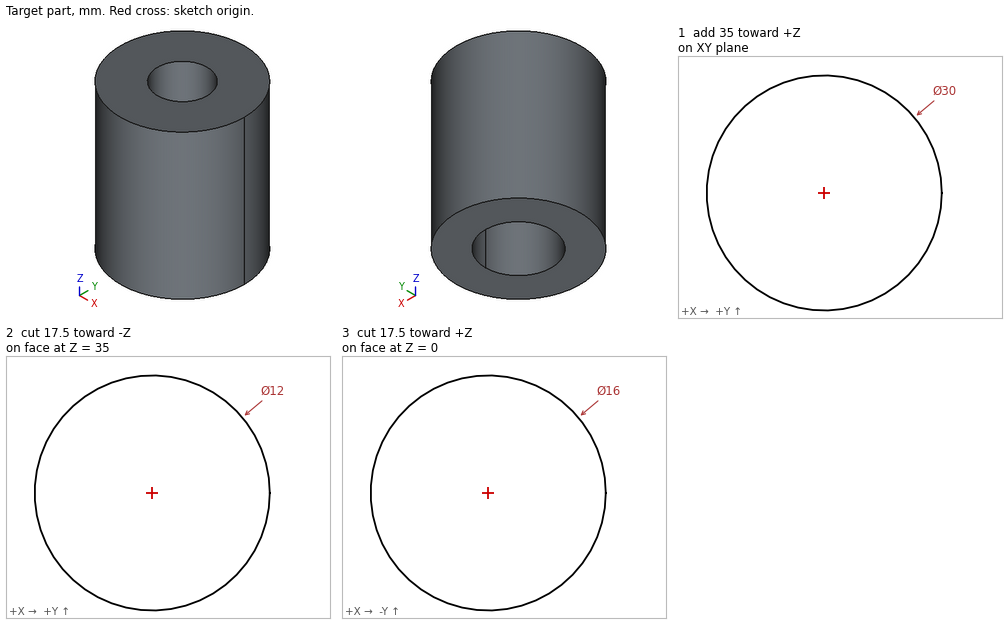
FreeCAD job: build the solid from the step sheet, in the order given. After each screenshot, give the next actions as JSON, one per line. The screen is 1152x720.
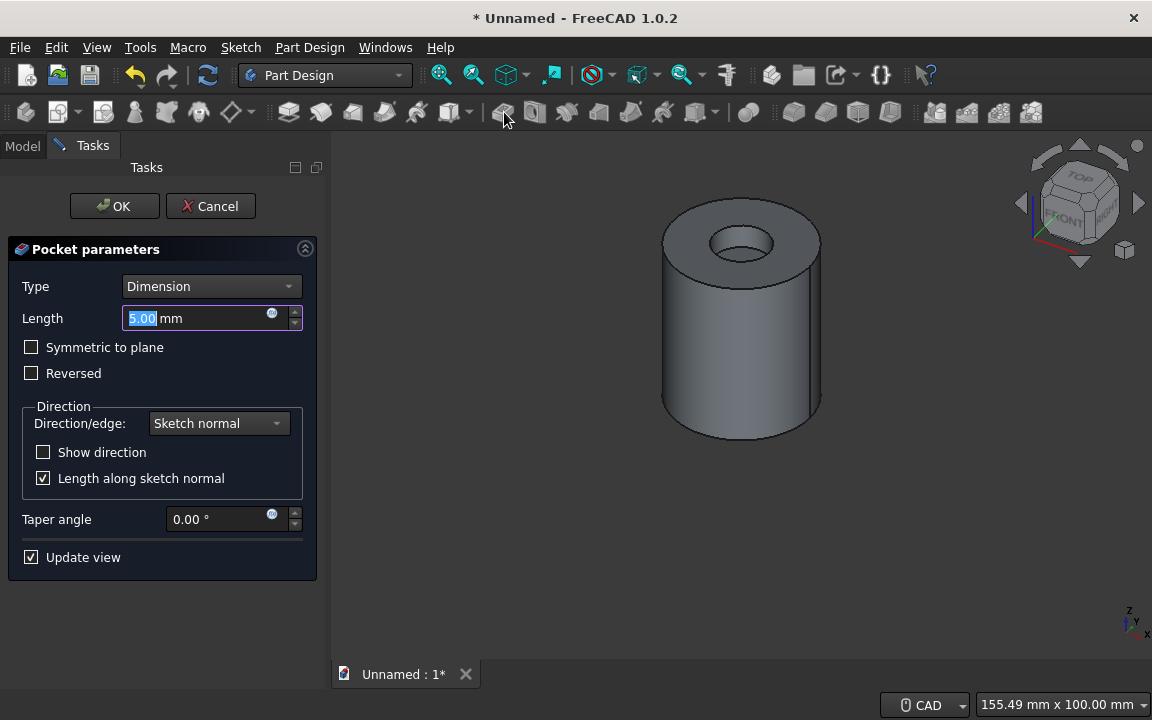
{"action": "type", "text": "17.5"}
{"action": "key", "text": "Tab"}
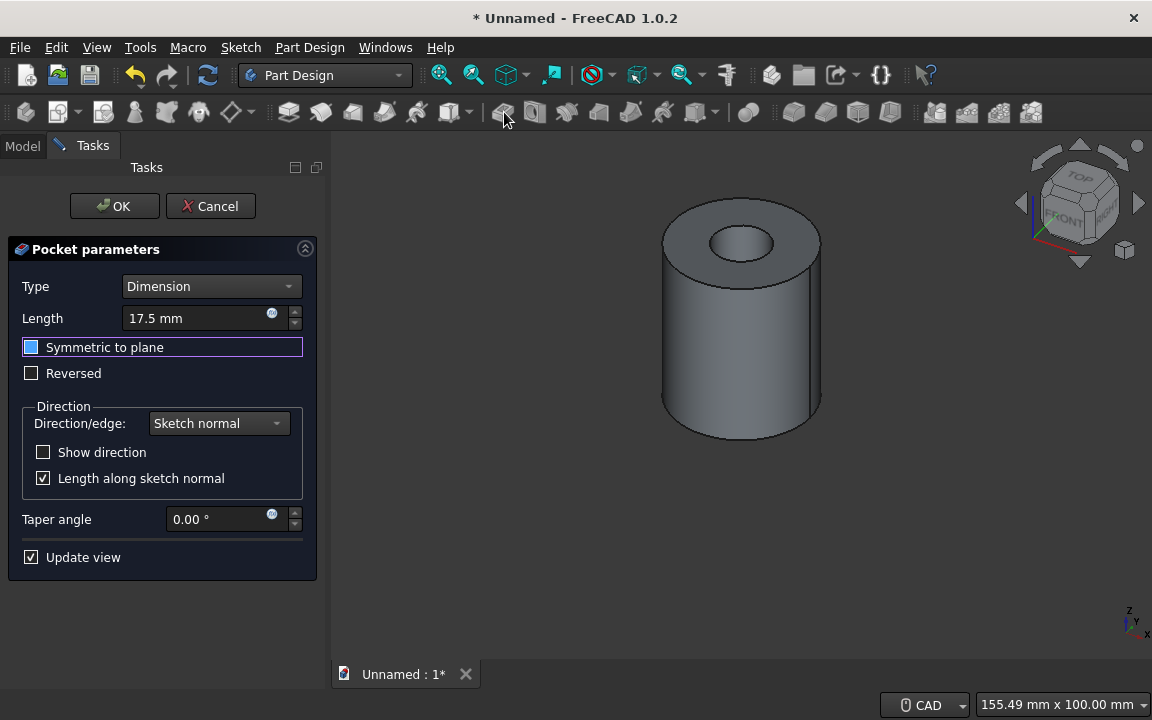
{"action": "left_click", "coordinate": [115, 206]}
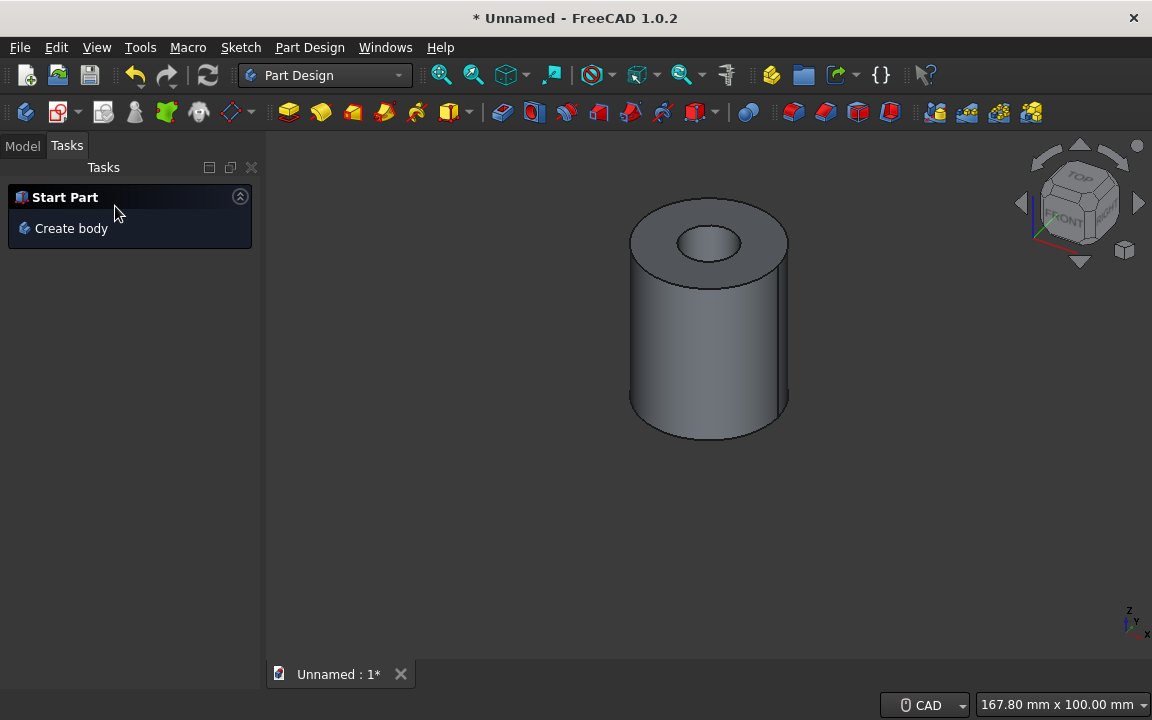
{"action": "key", "text": "5"}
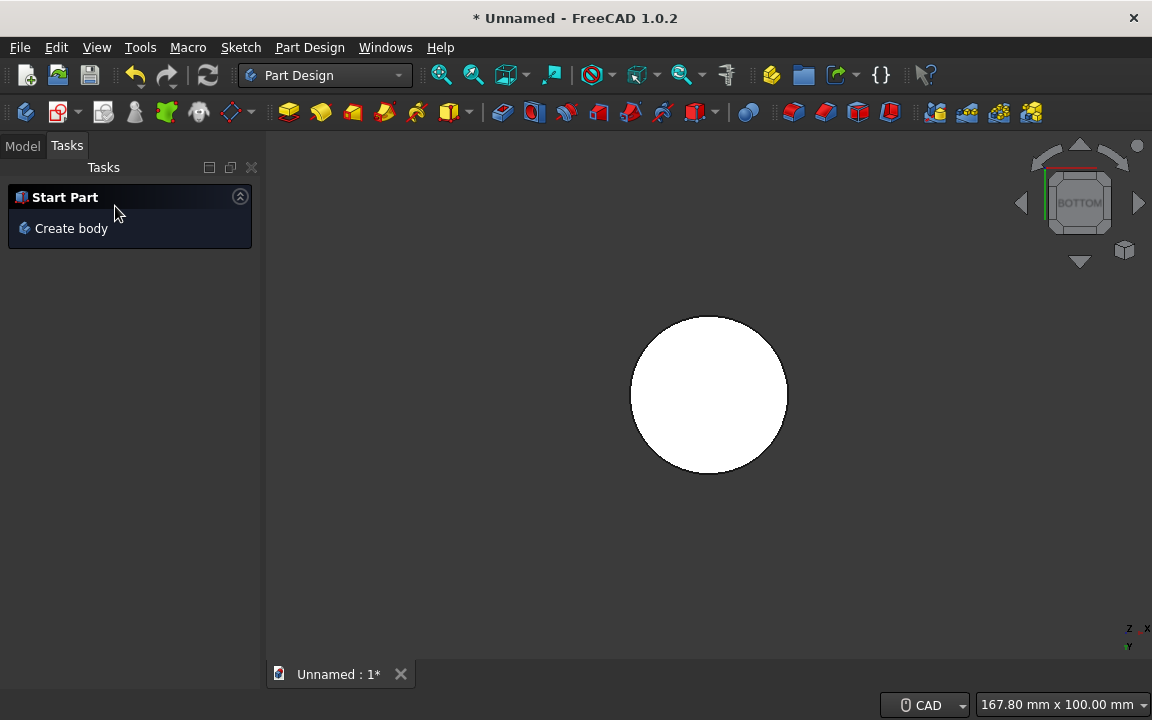
{"action": "left_click", "coordinate": [442, 76]}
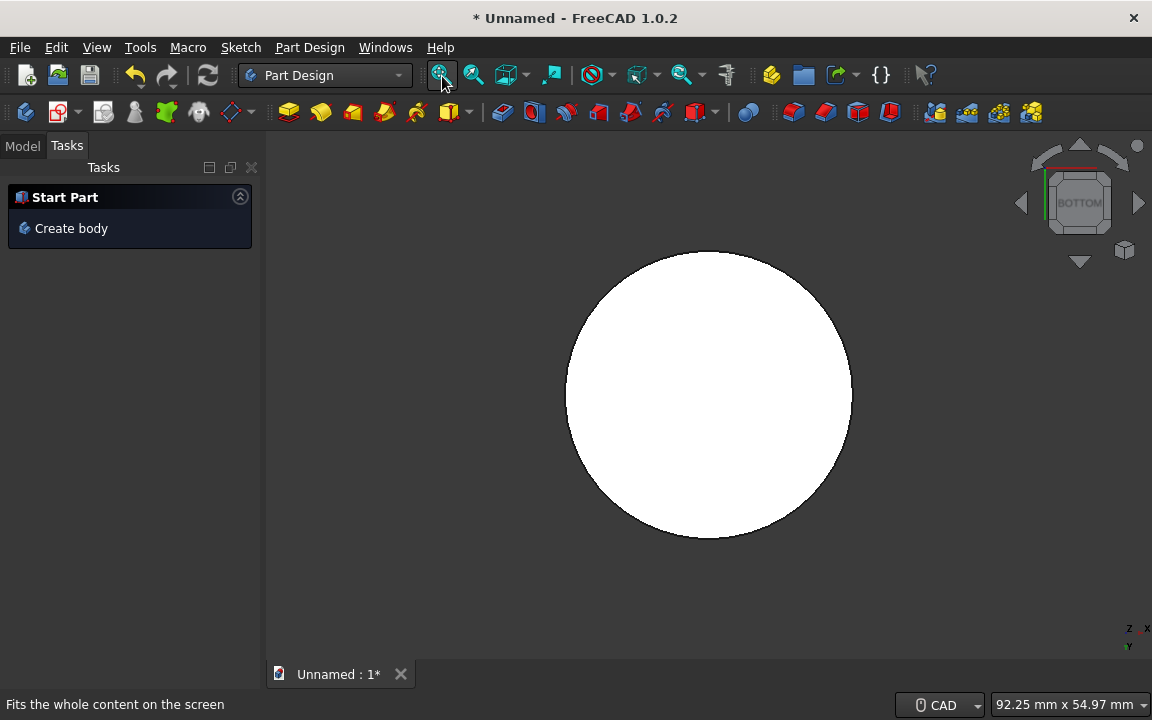
{"action": "left_click", "coordinate": [709, 394]}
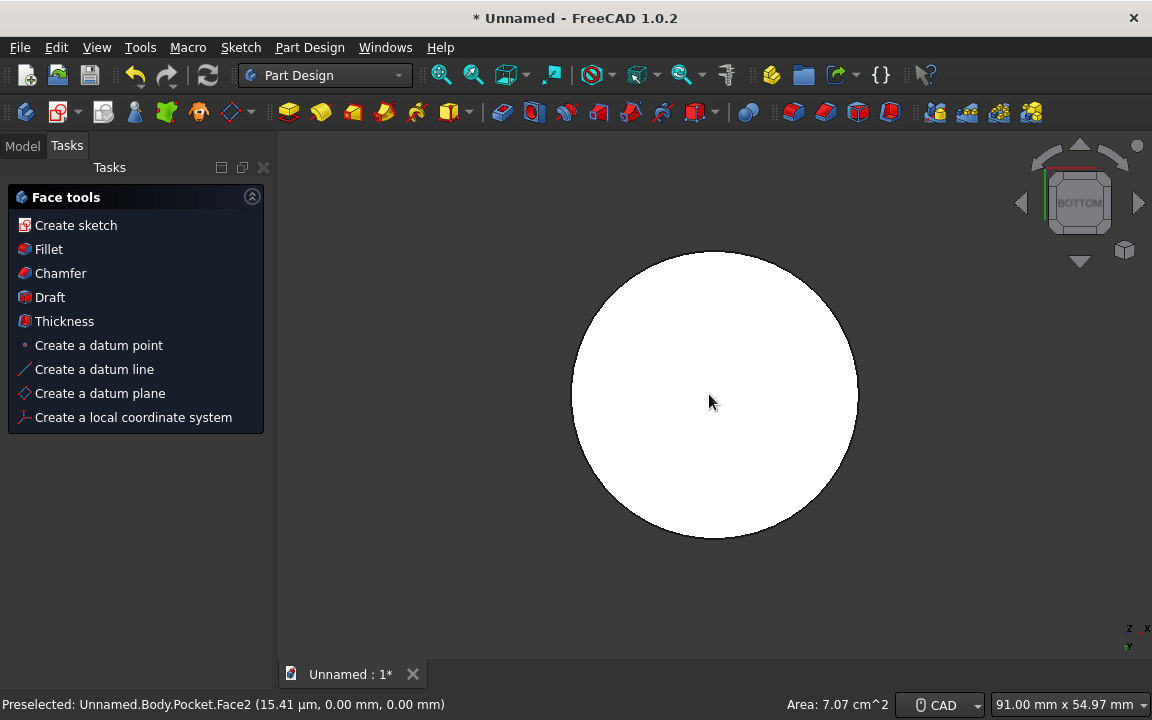
{"action": "left_click", "coordinate": [58, 112]}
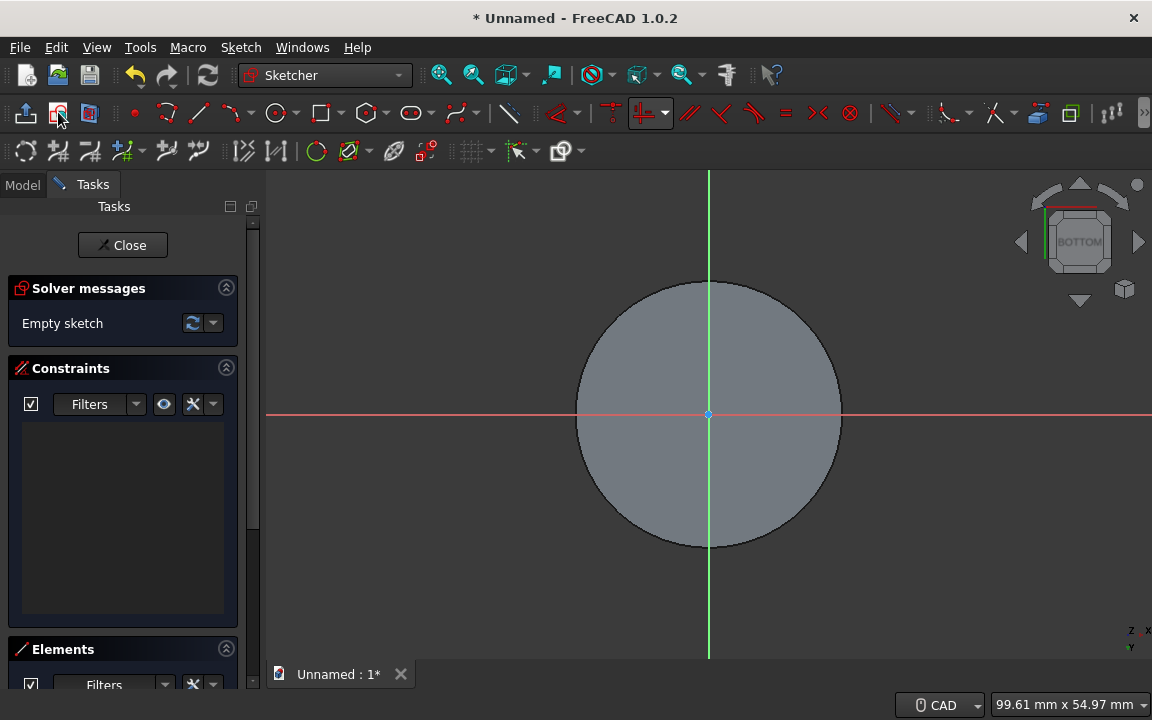
{"action": "scroll", "coordinate": [765, 414], "scroll_direction": "up", "scroll_amount": 4}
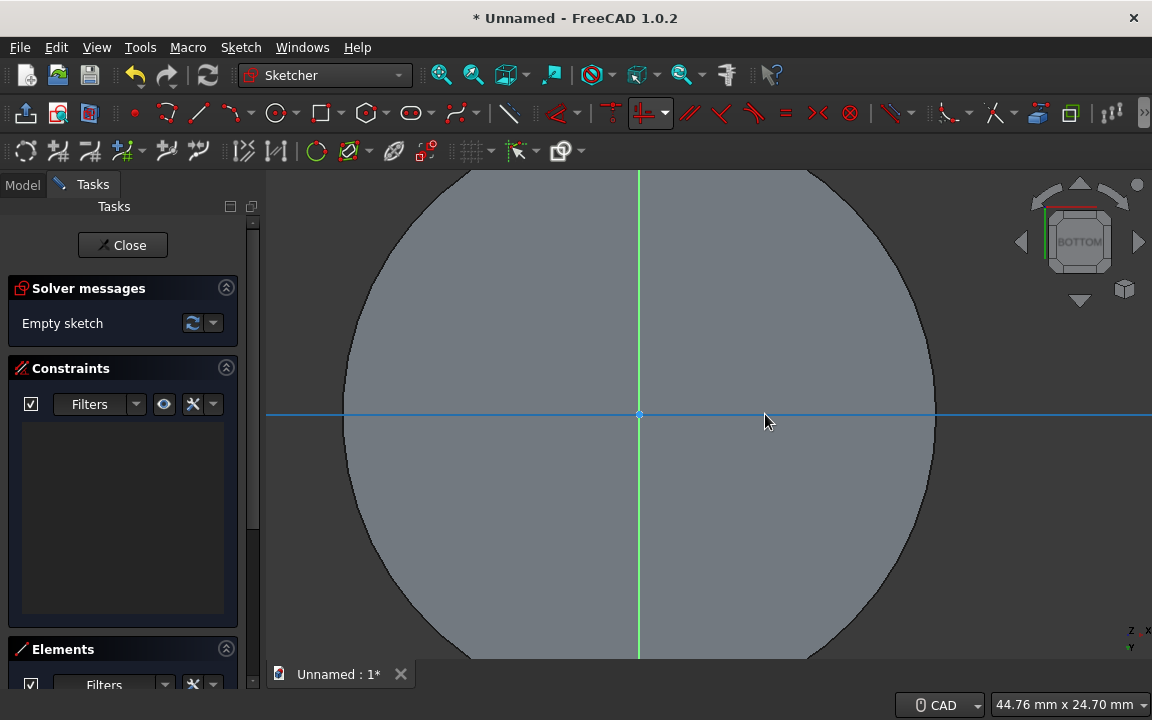
{"action": "left_click", "coordinate": [276, 114]}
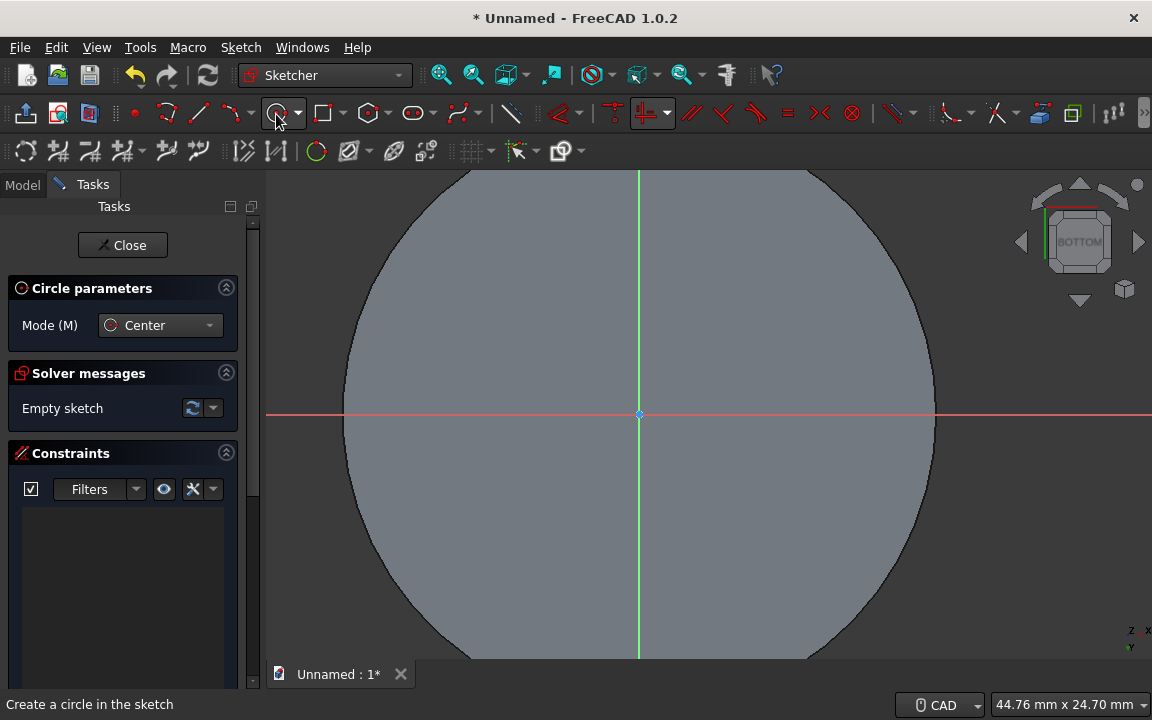
{"action": "left_click", "coordinate": [639, 414]}
{"action": "left_click", "coordinate": [751, 303]}
{"action": "key", "text": "Escape"}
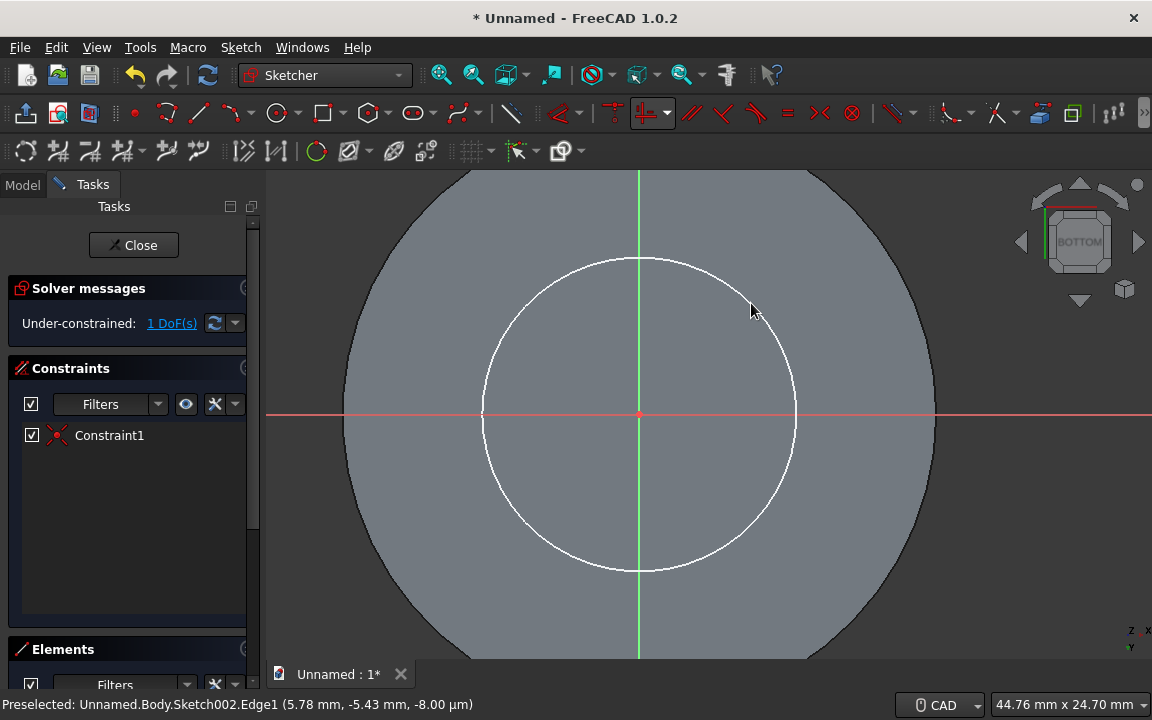
{"action": "key", "text": "d"}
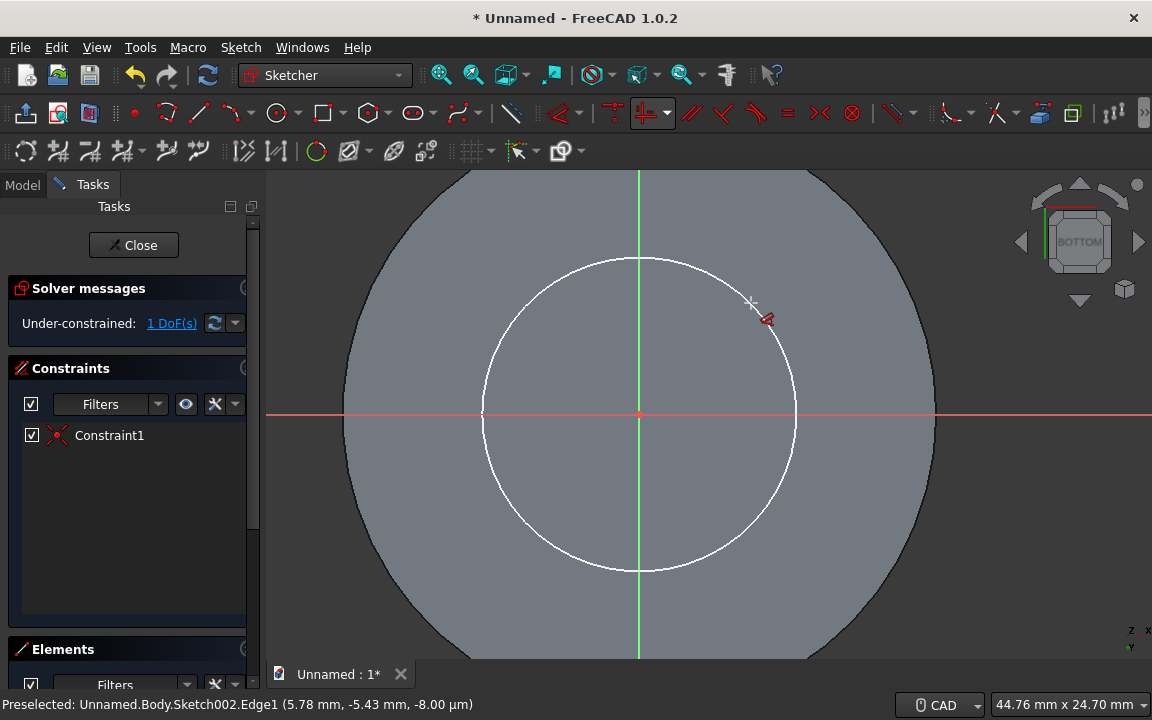
{"action": "left_click", "coordinate": [750, 303]}
{"action": "left_click", "coordinate": [773, 280]}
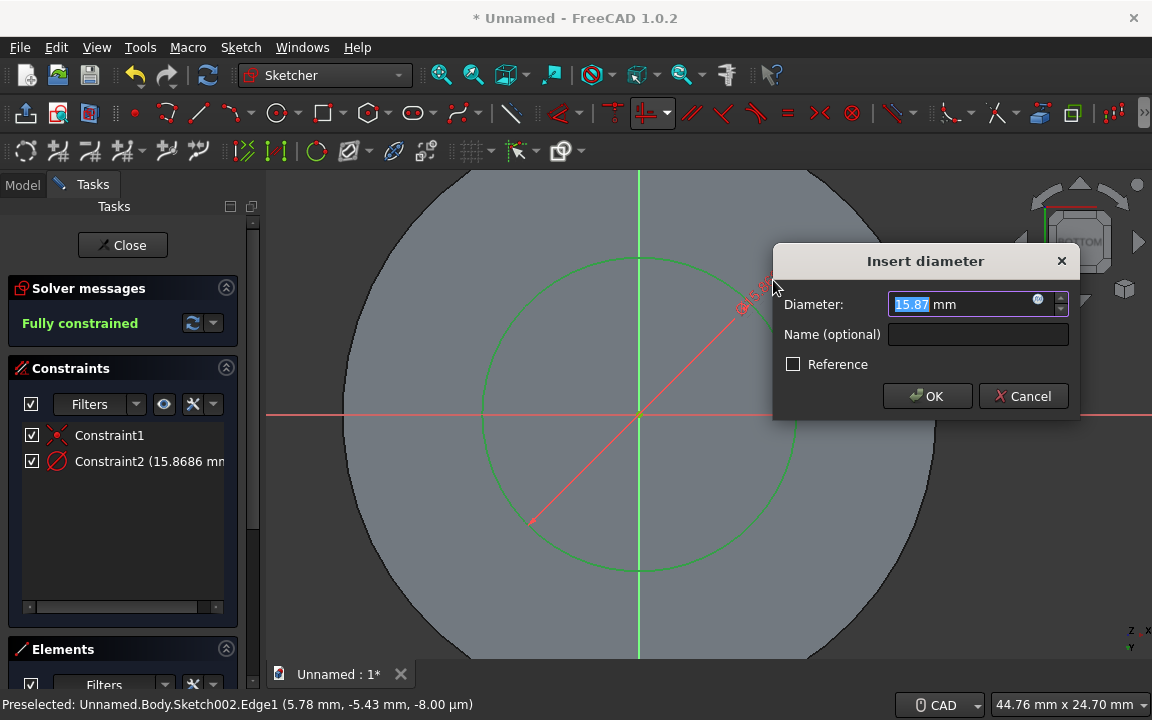
{"action": "type", "text": "16"}
{"action": "key", "text": "Return"}
{"action": "key", "text": "Escape"}